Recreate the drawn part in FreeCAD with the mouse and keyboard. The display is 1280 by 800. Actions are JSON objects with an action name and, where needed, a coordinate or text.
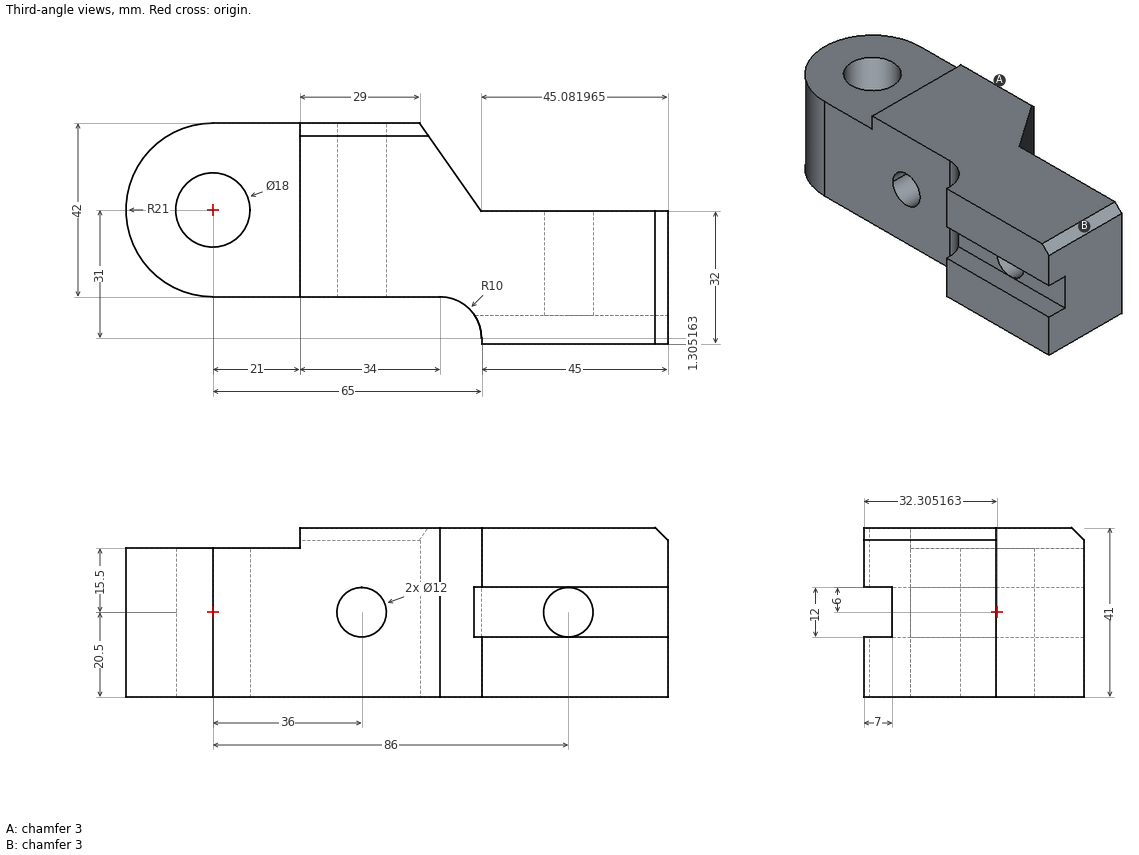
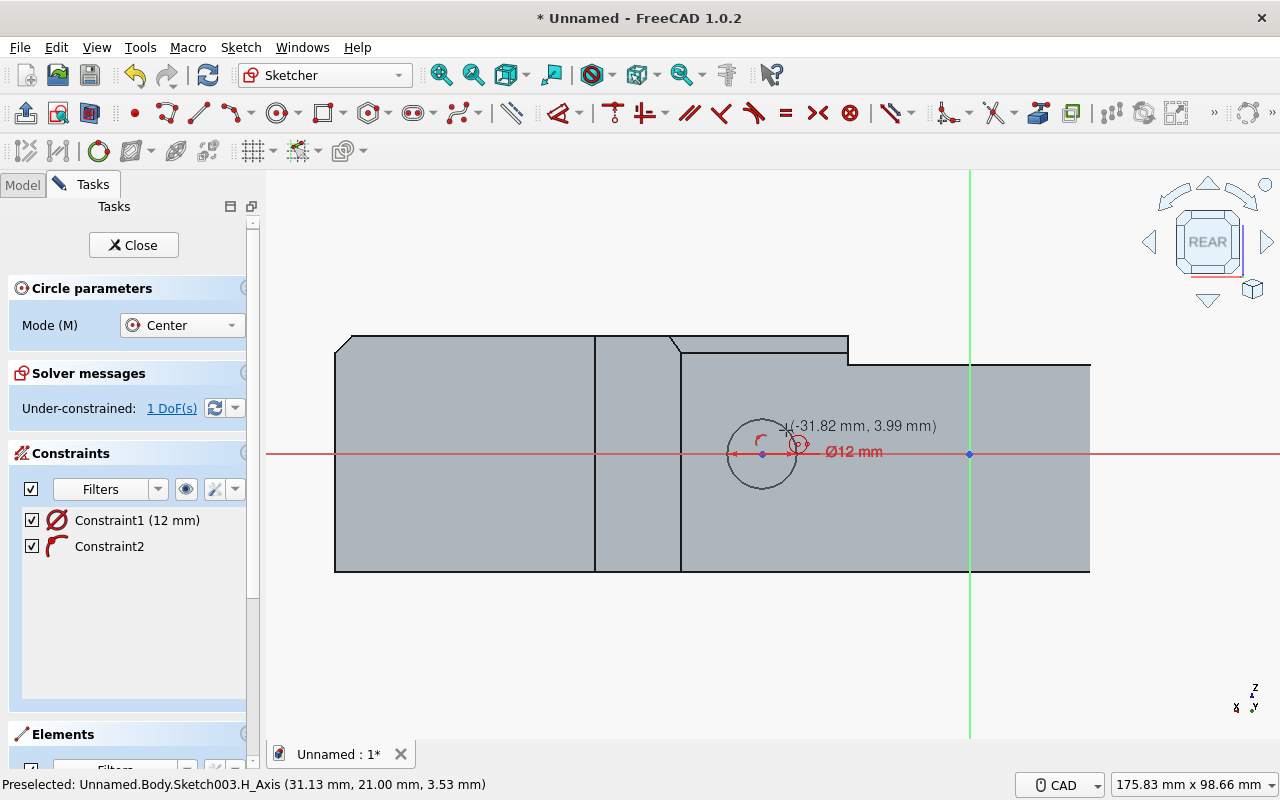
{"action": "left_click", "coordinate": [474, 454]}
{"action": "mouse_move", "coordinate": [498, 430]}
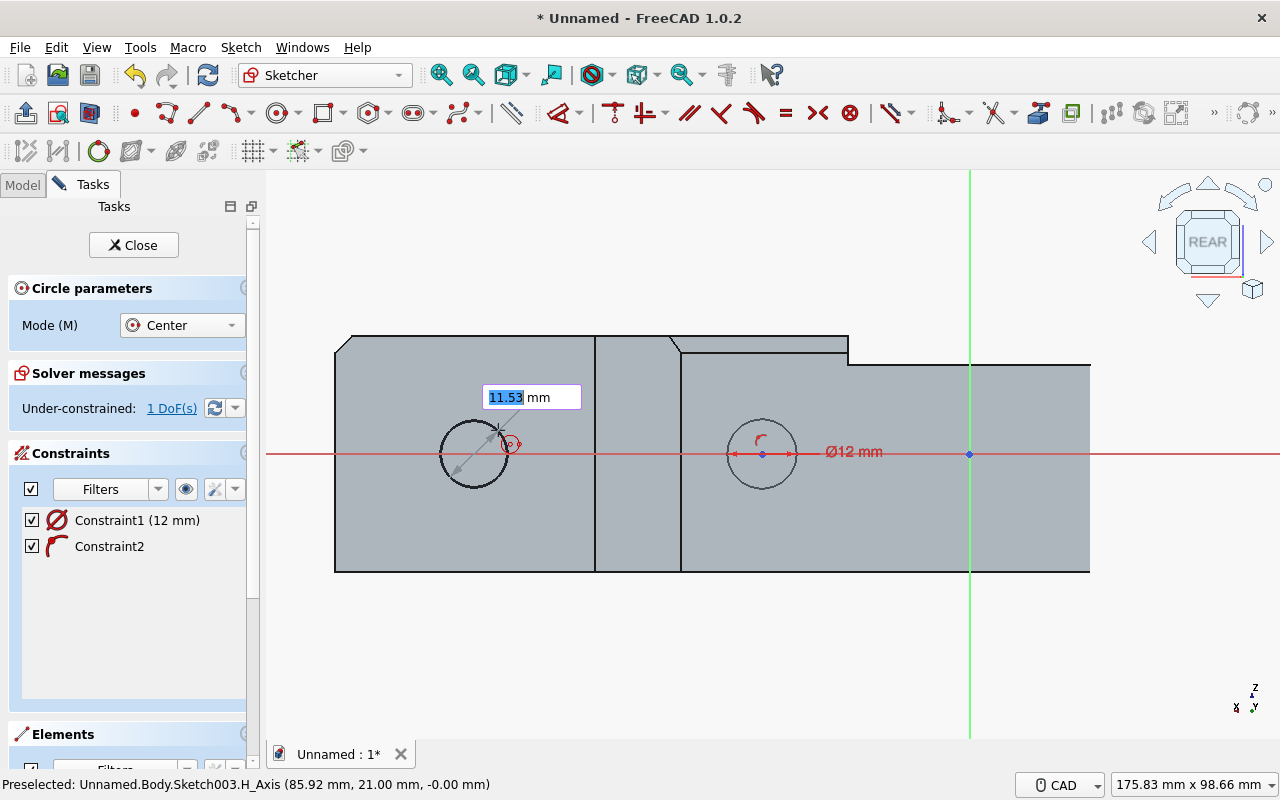
{"action": "type", "text": "12"}
{"action": "key", "text": "Return"}
{"action": "key", "text": "Escape"}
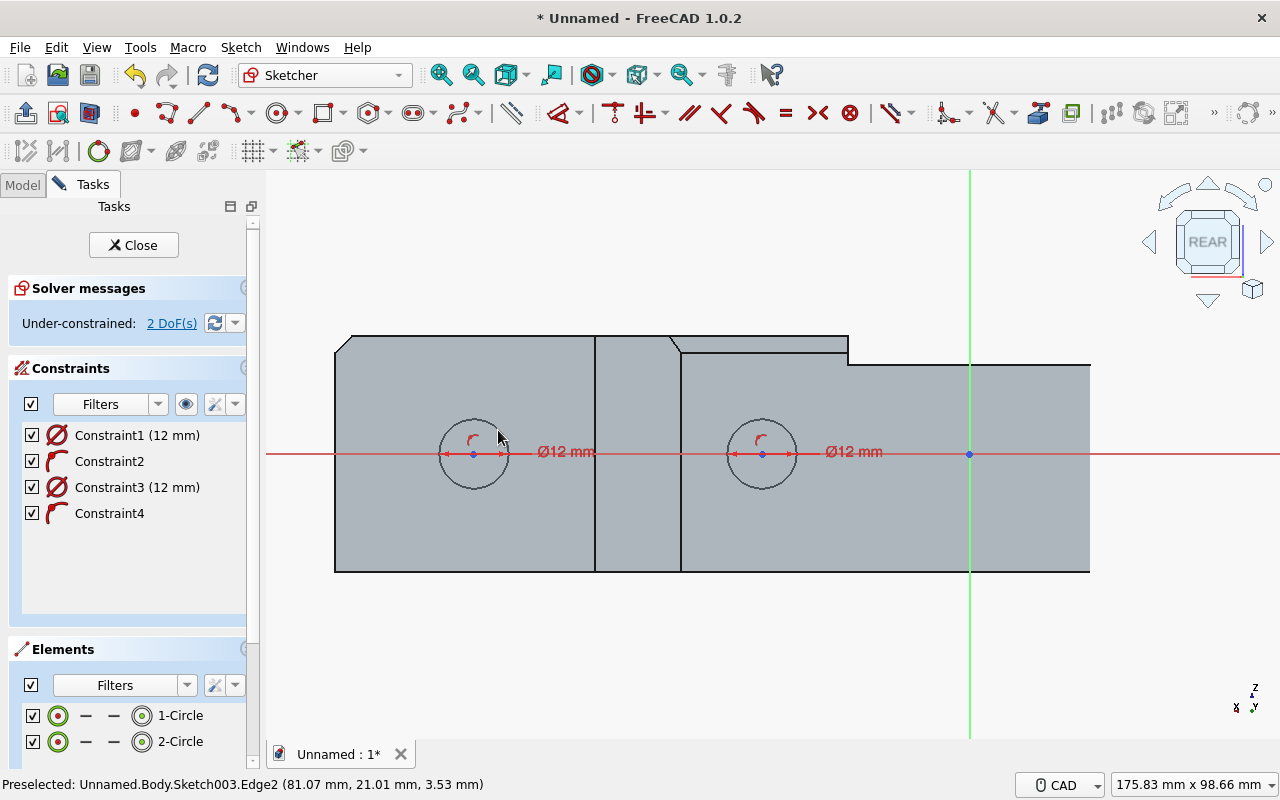
{"action": "left_click", "coordinate": [558, 114]}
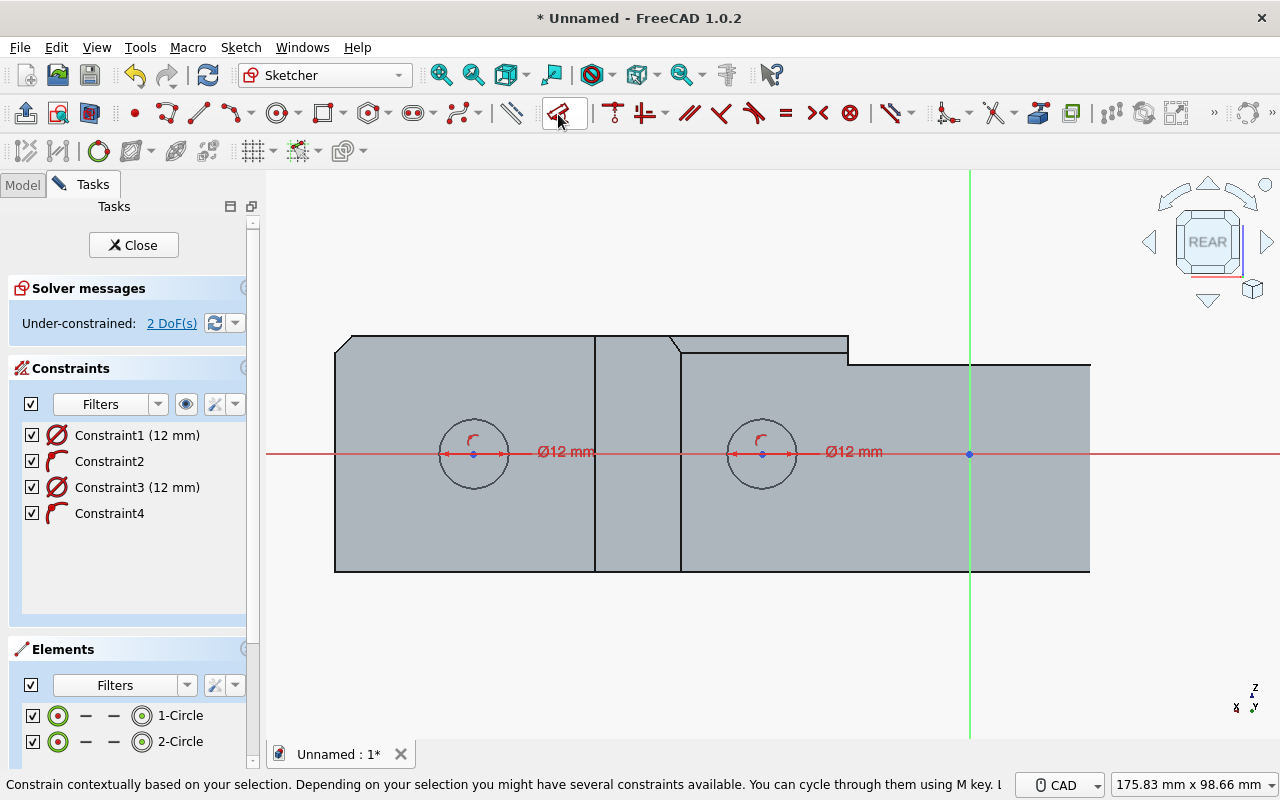
{"action": "left_click", "coordinate": [762, 454]}
{"action": "left_click", "coordinate": [866, 488]}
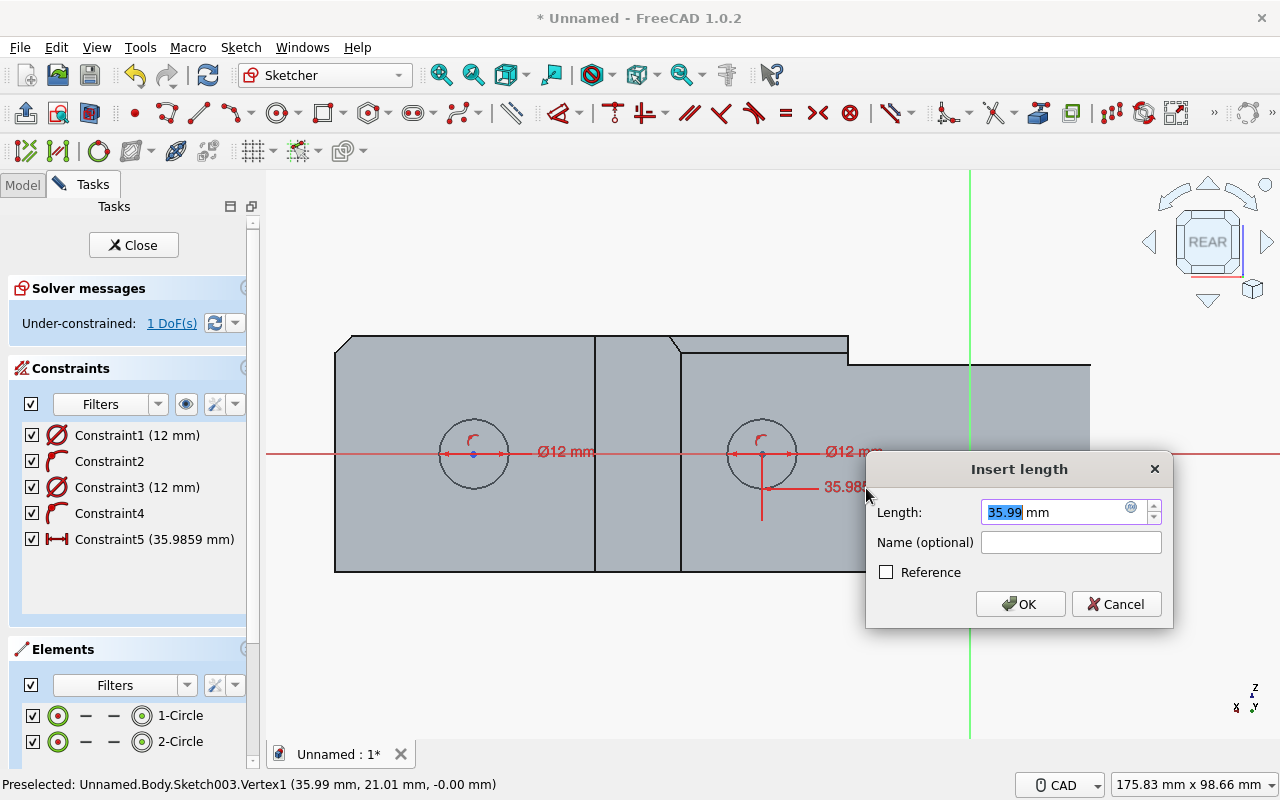
{"action": "type", "text": "36"}
{"action": "key", "text": "Return"}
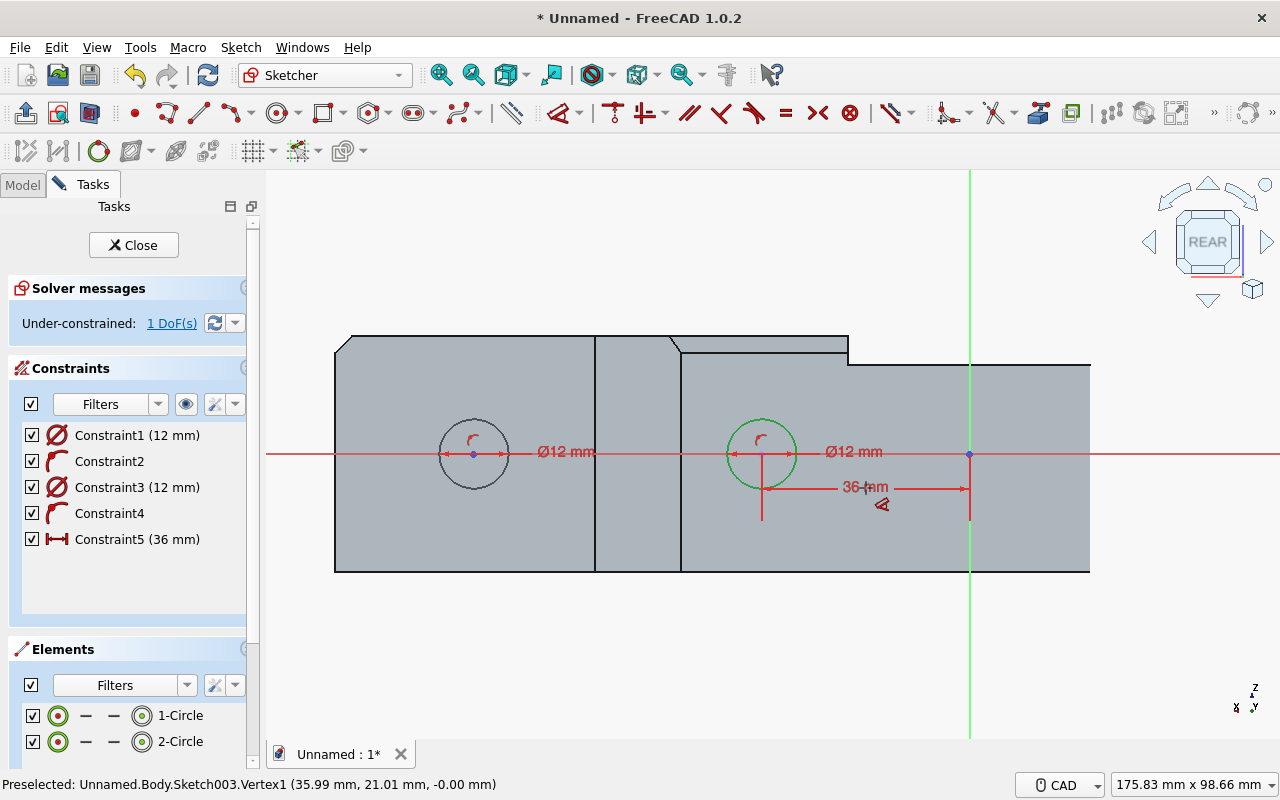
{"action": "left_click", "coordinate": [474, 454]}
{"action": "left_click", "coordinate": [722, 488]}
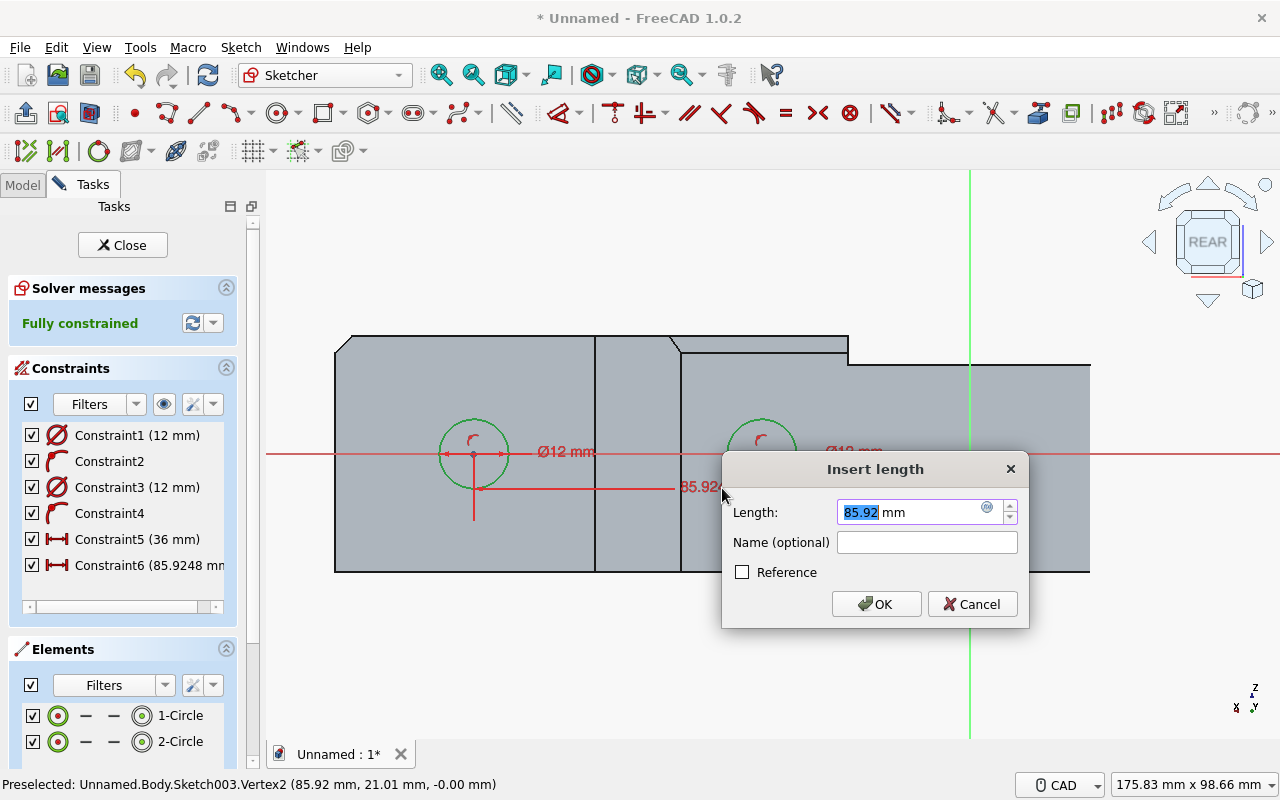
{"action": "type", "text": "86"}
{"action": "key", "text": "Return"}
{"action": "key", "text": "Escape"}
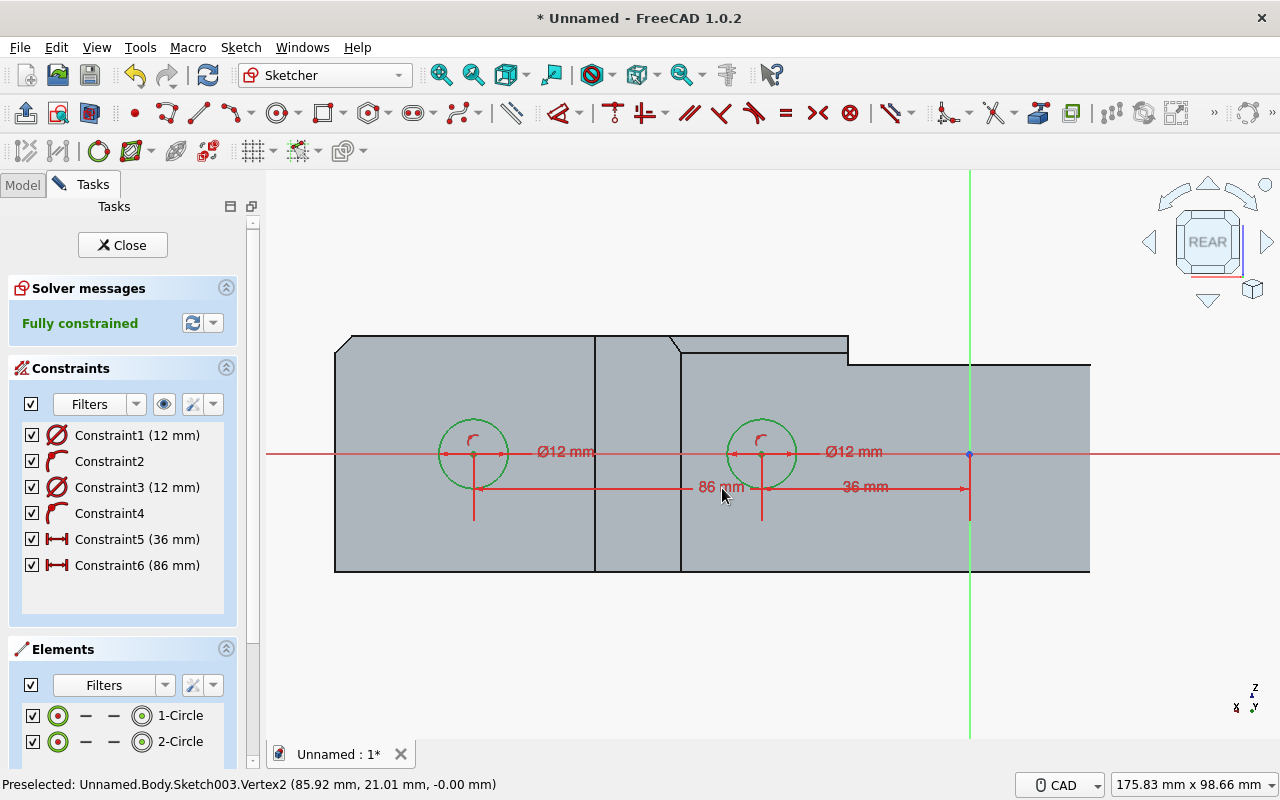
{"action": "left_click", "coordinate": [123, 245]}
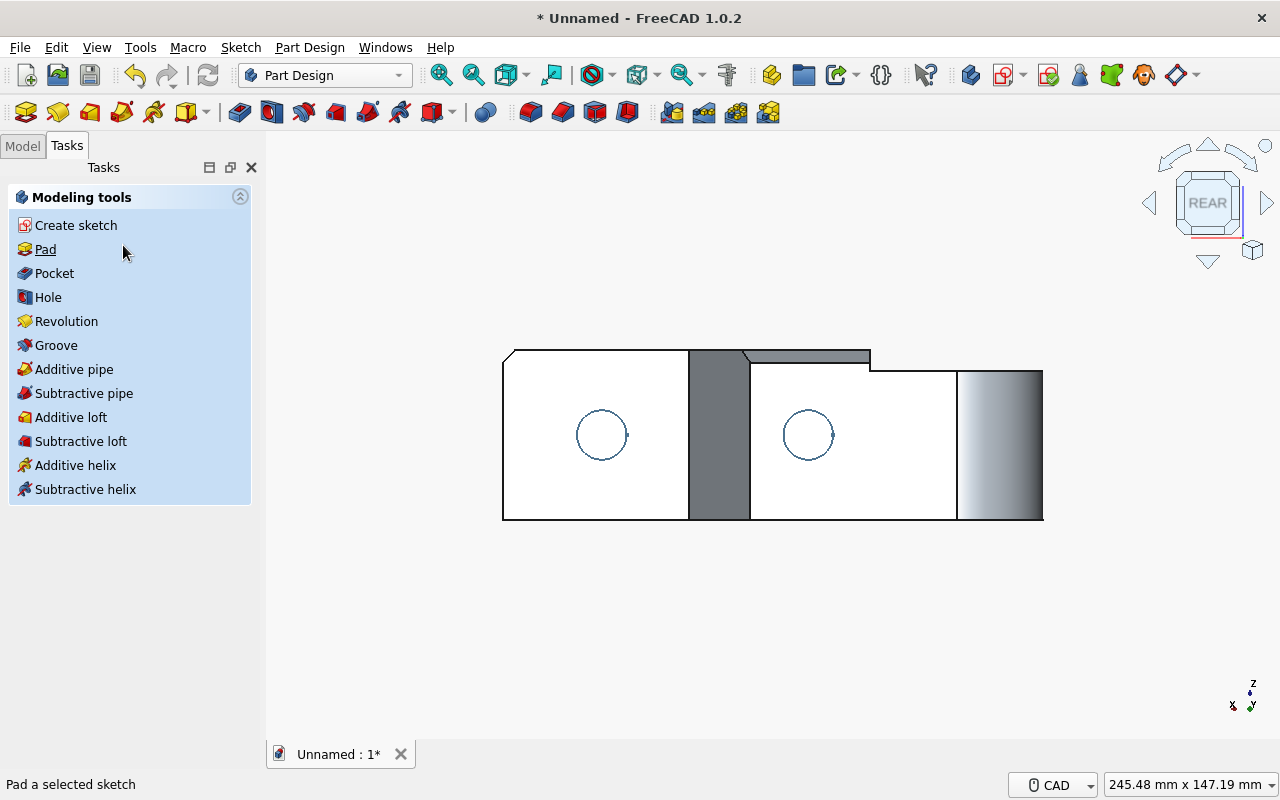
{"action": "left_click", "coordinate": [240, 112]}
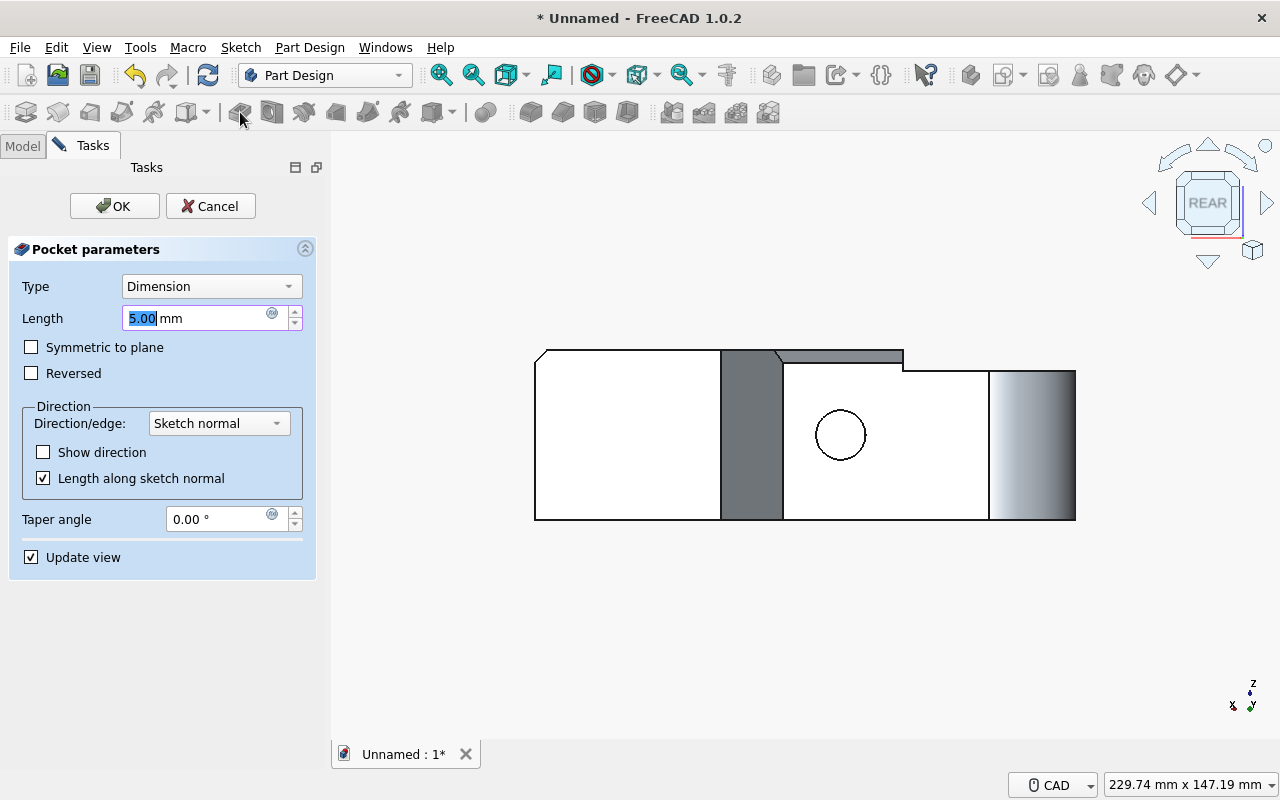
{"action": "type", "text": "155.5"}
{"action": "key", "text": "Tab"}